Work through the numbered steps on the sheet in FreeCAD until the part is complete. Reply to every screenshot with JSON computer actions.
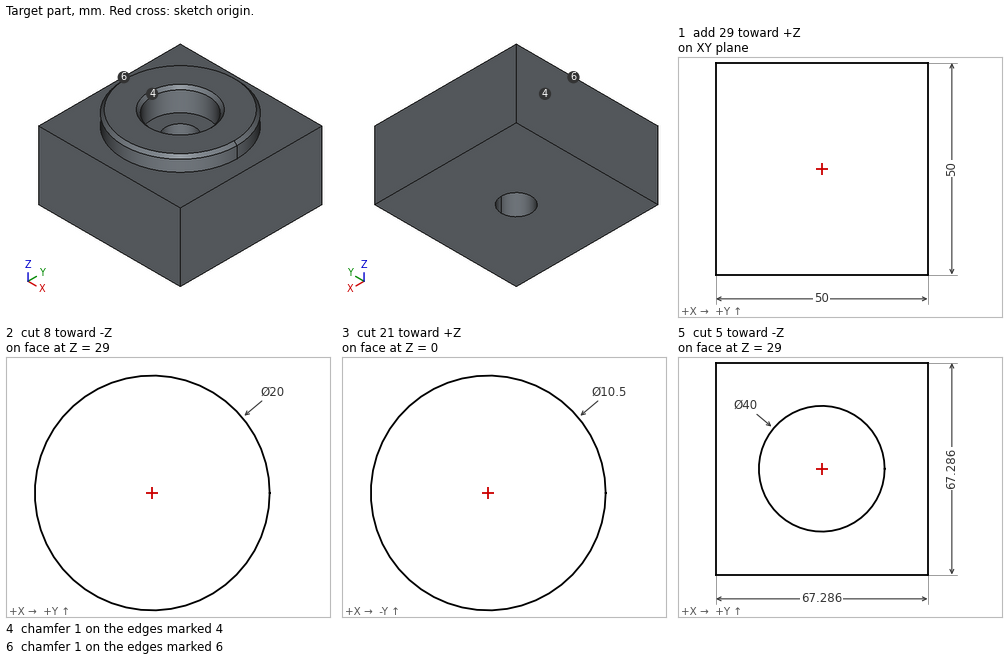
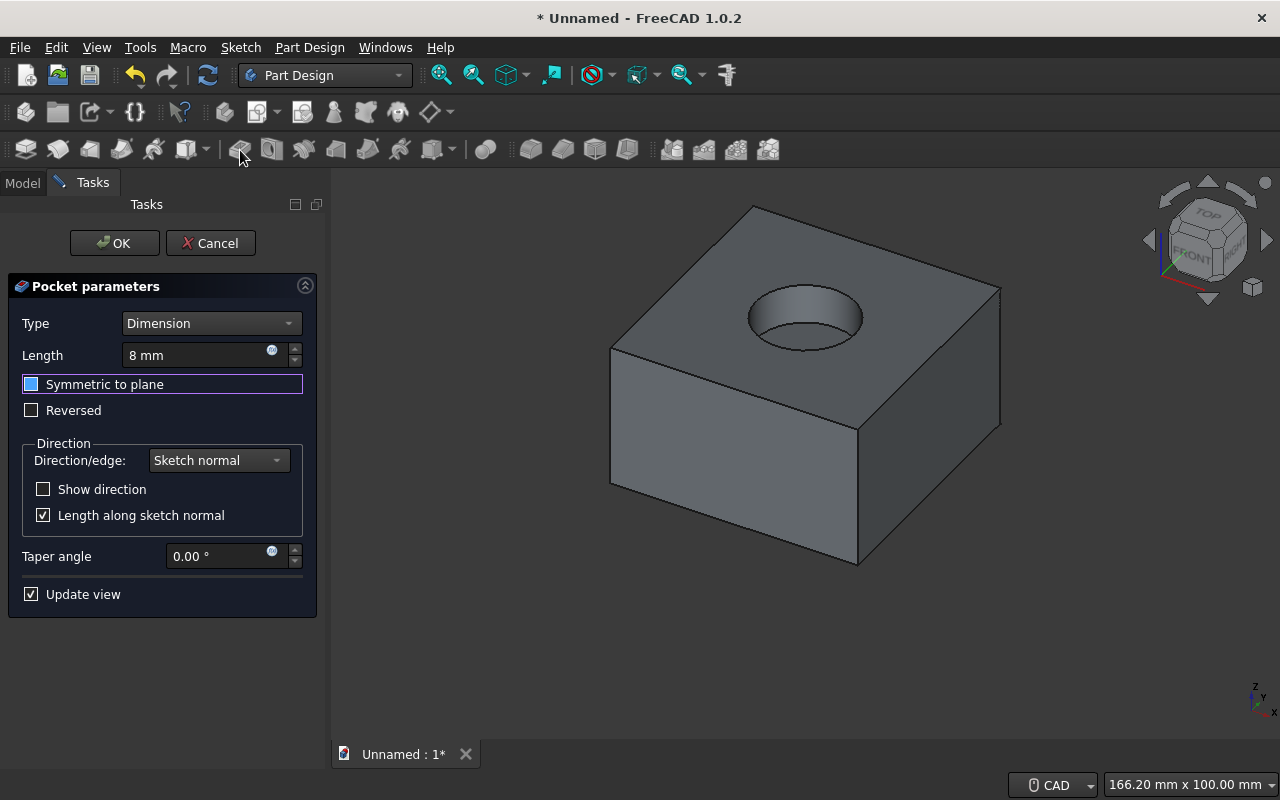
{"action": "left_click", "coordinate": [115, 243]}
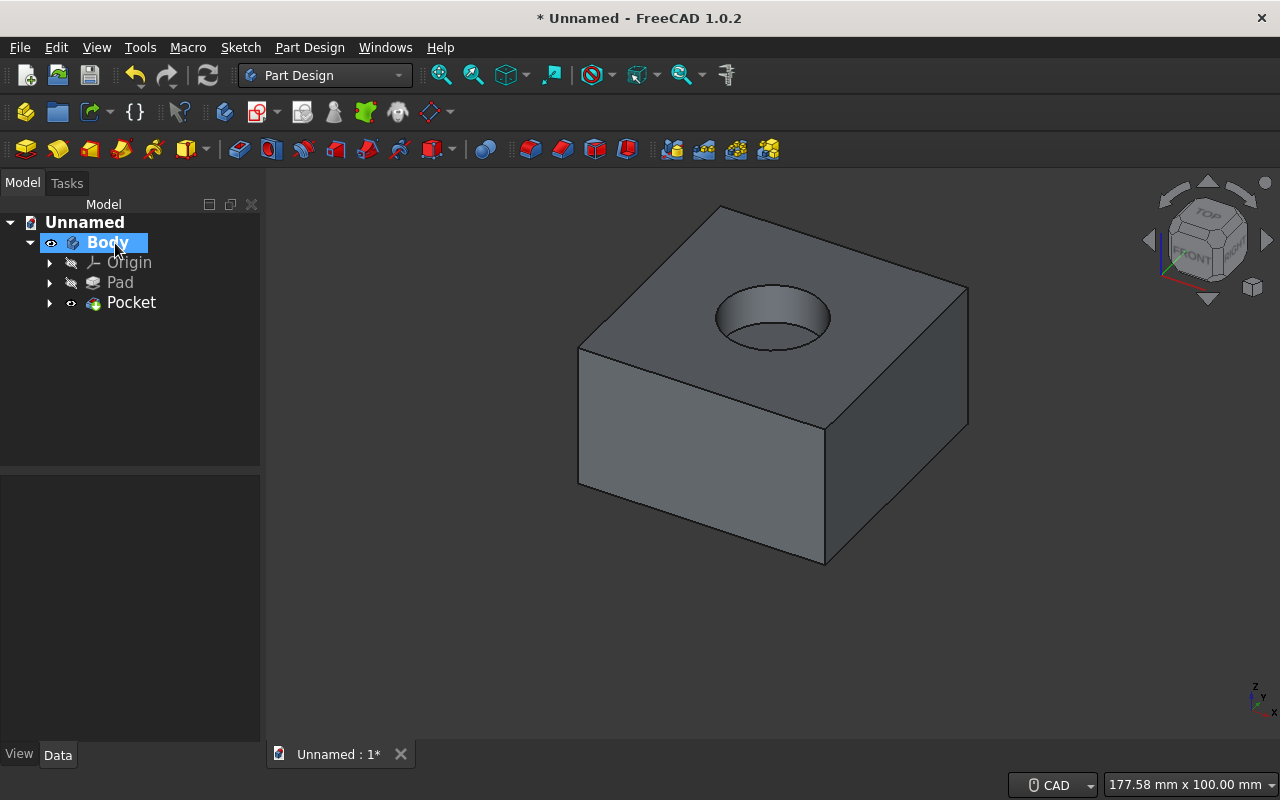
{"action": "key", "text": "5"}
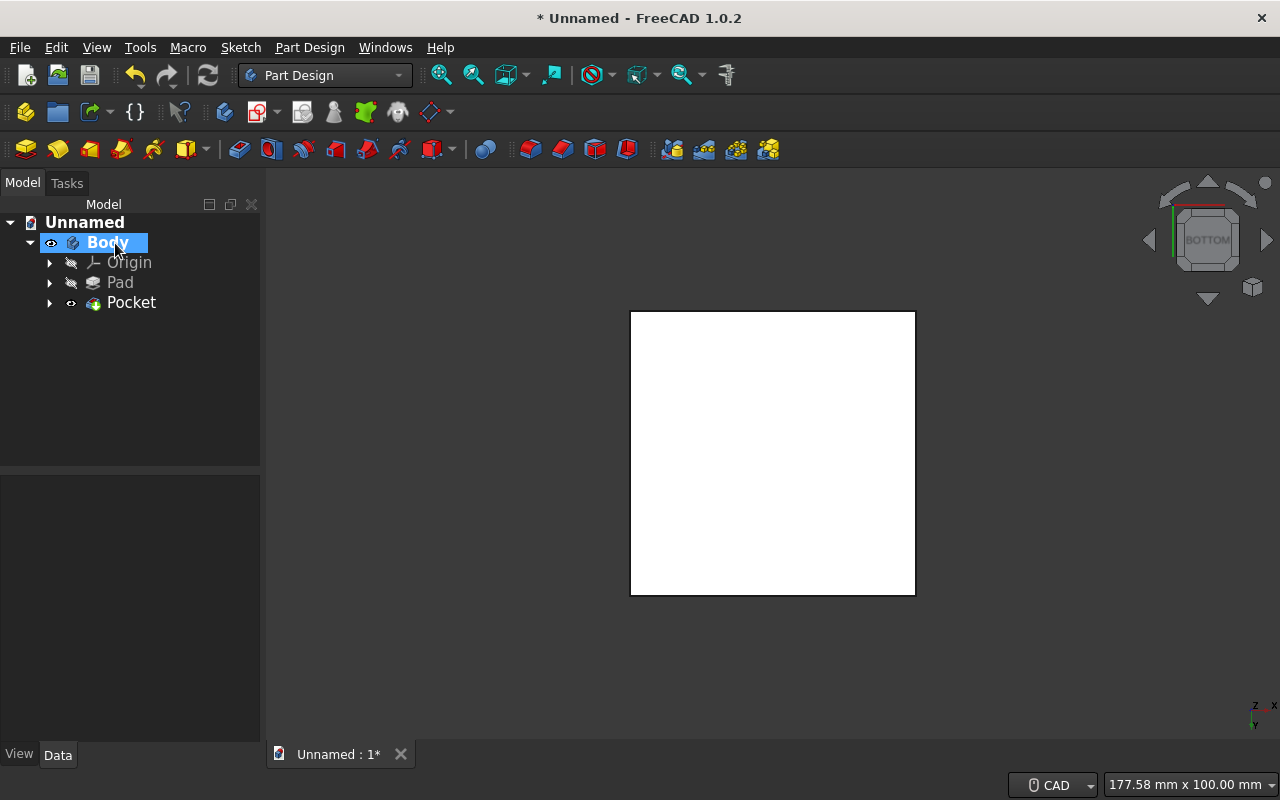
{"action": "left_click", "coordinate": [773, 452]}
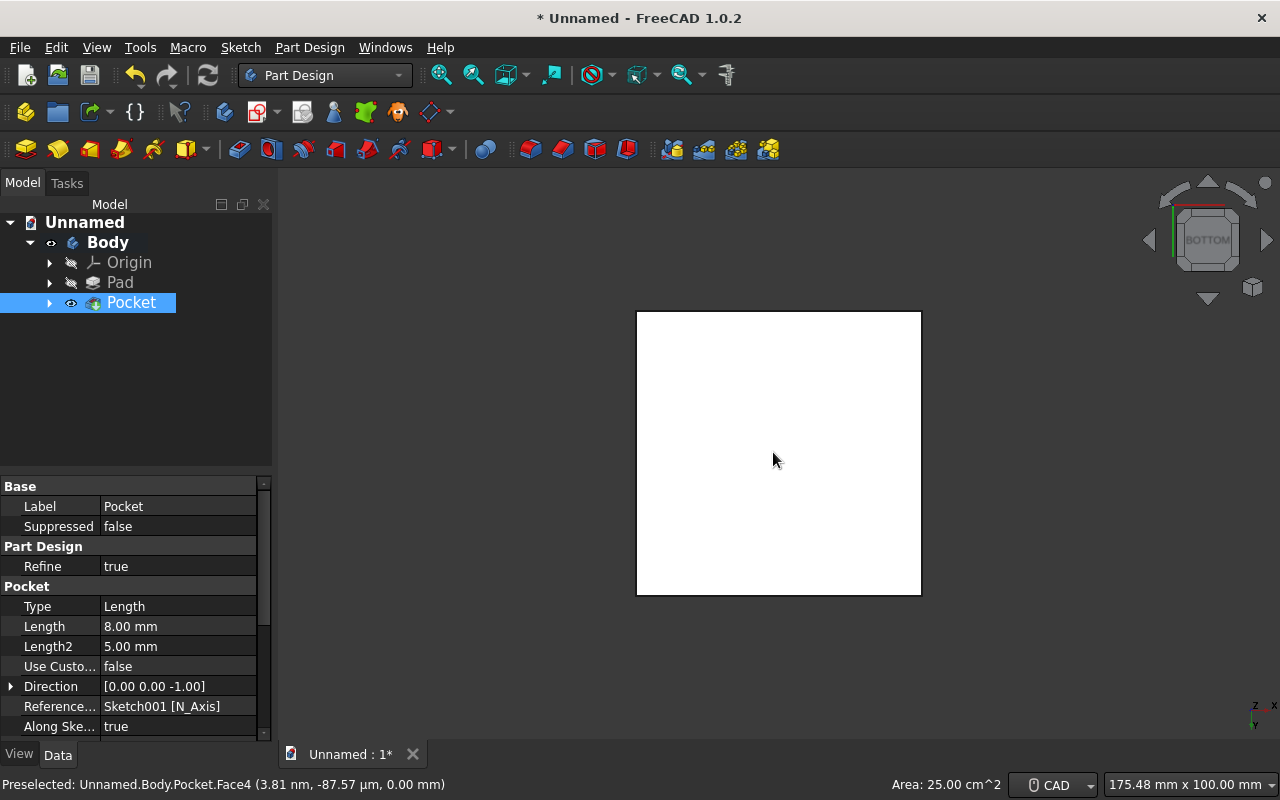
{"action": "left_click", "coordinate": [258, 112]}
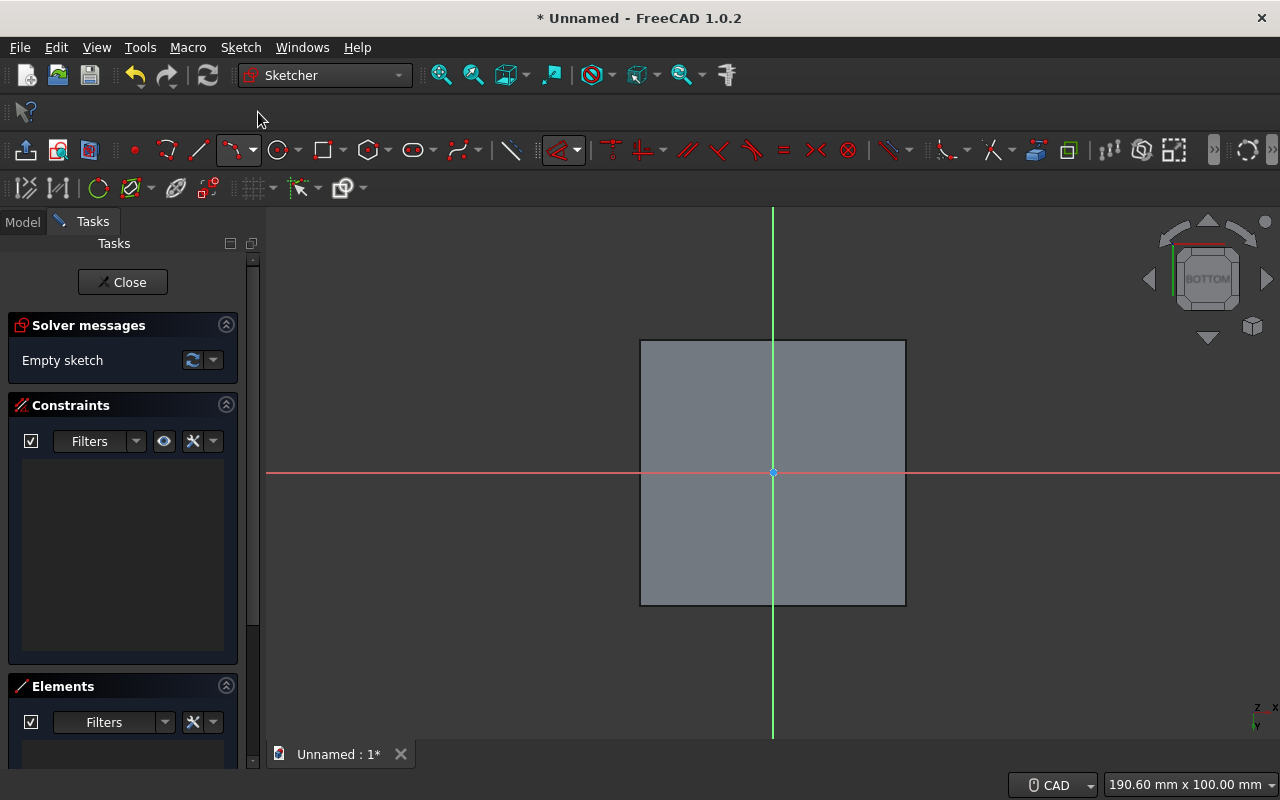
{"action": "scroll", "coordinate": [787, 473], "scroll_direction": "up", "scroll_amount": 9}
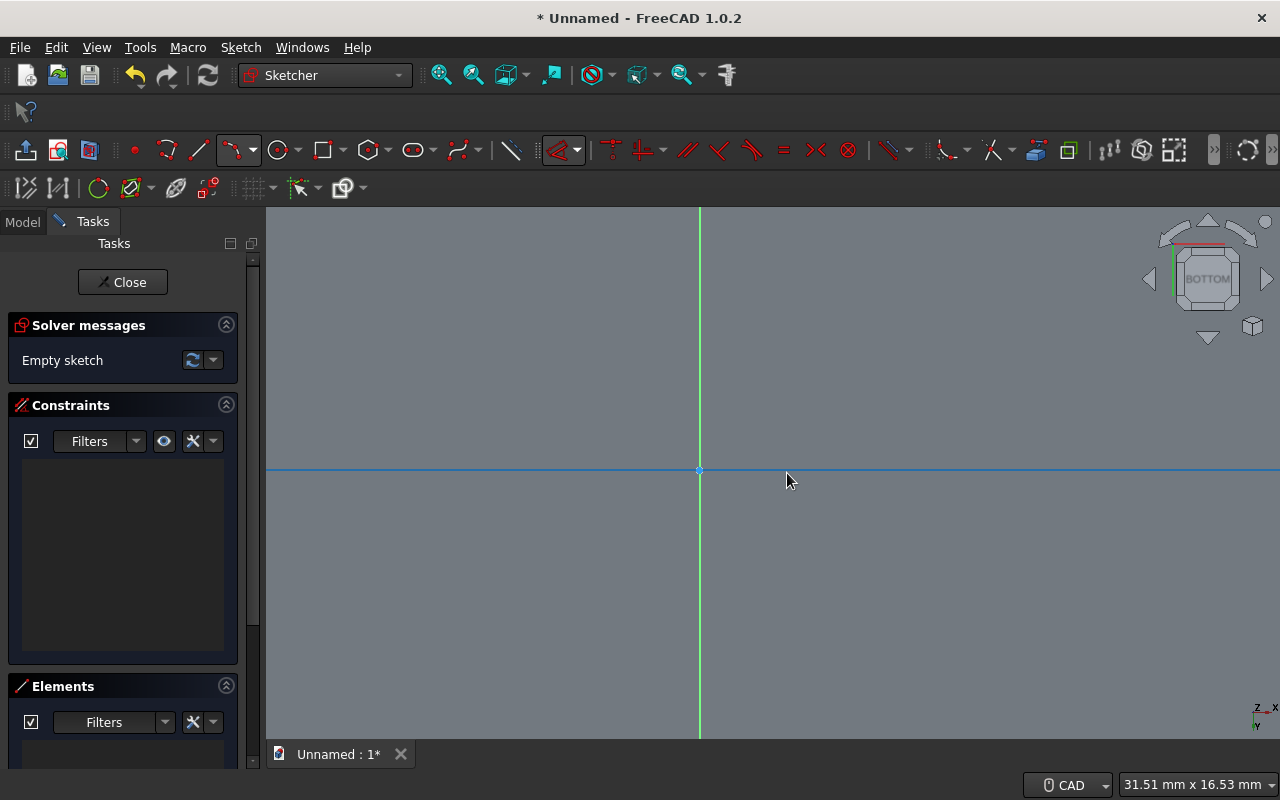
{"action": "left_click", "coordinate": [278, 150]}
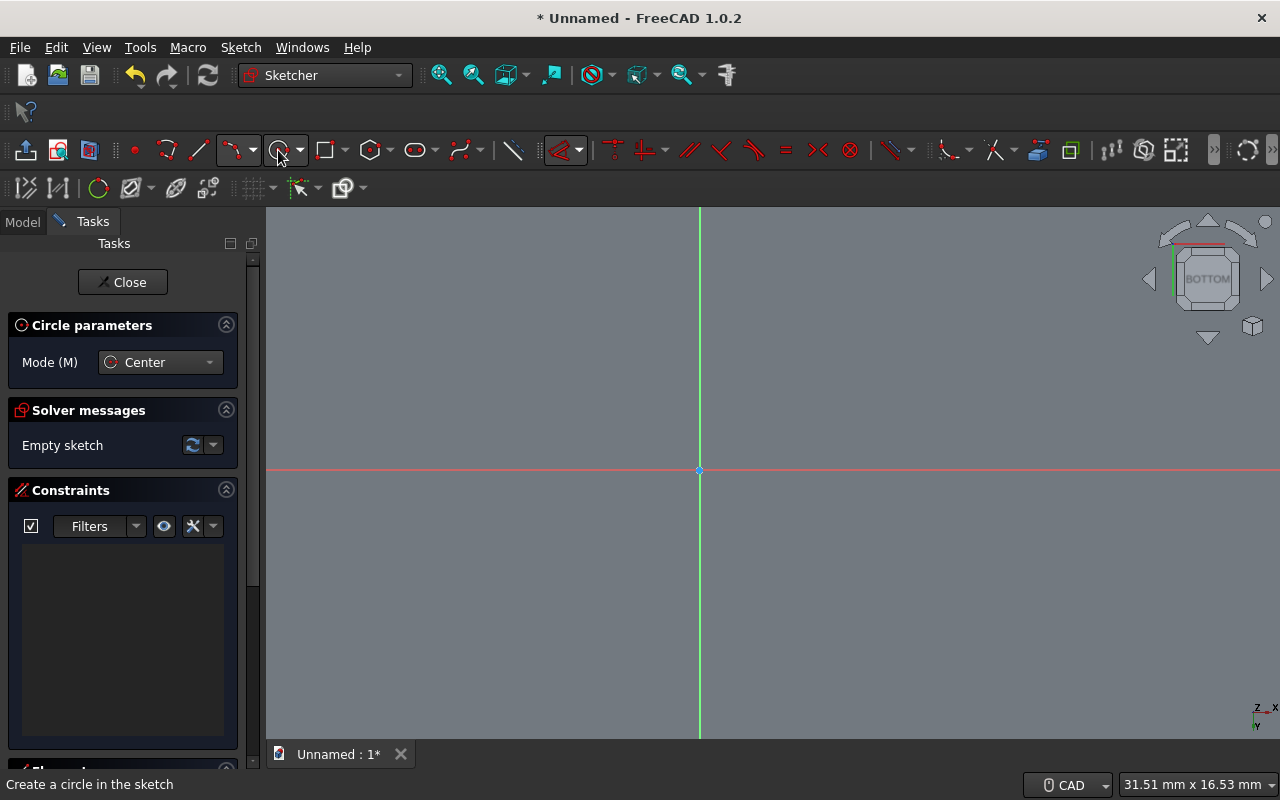
{"action": "left_click", "coordinate": [700, 470]}
{"action": "mouse_move", "coordinate": [819, 351]}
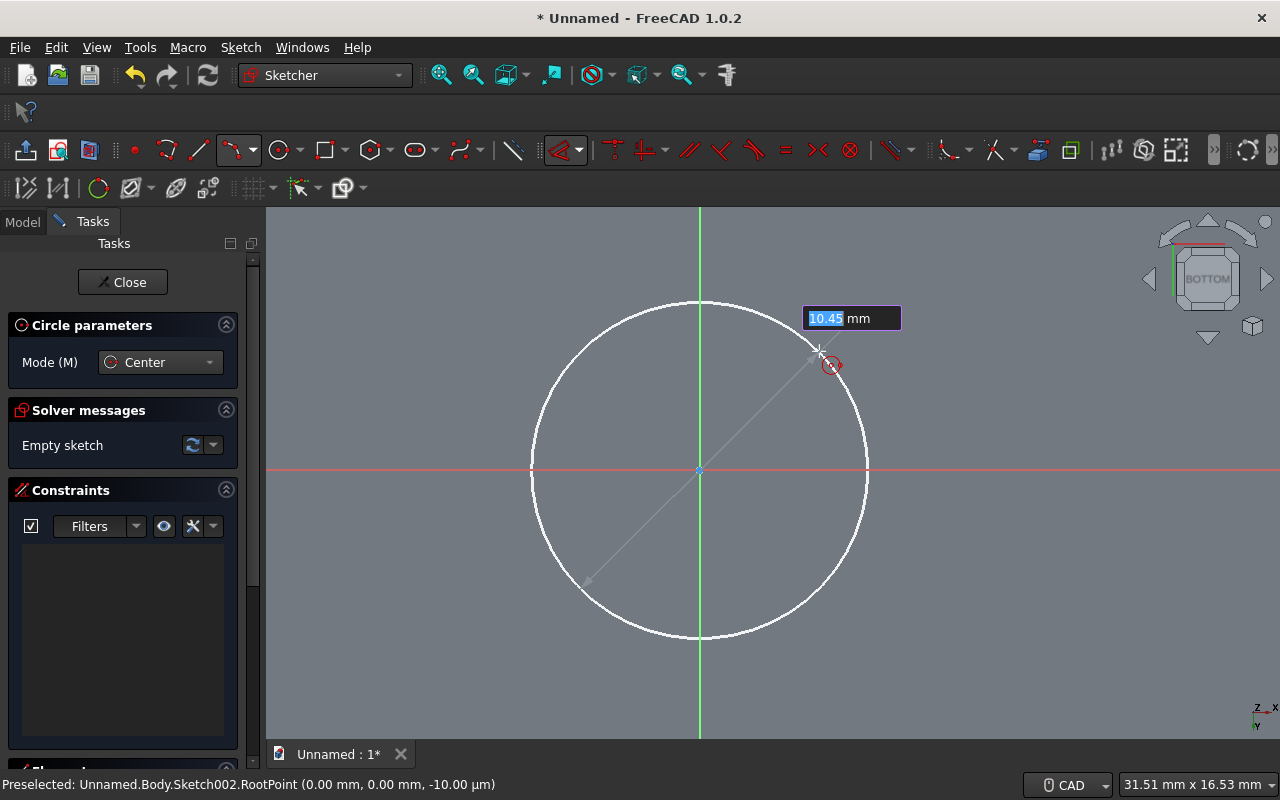
{"action": "type", "text": "10.5"}
{"action": "key", "text": "Return"}
{"action": "key", "text": "Escape"}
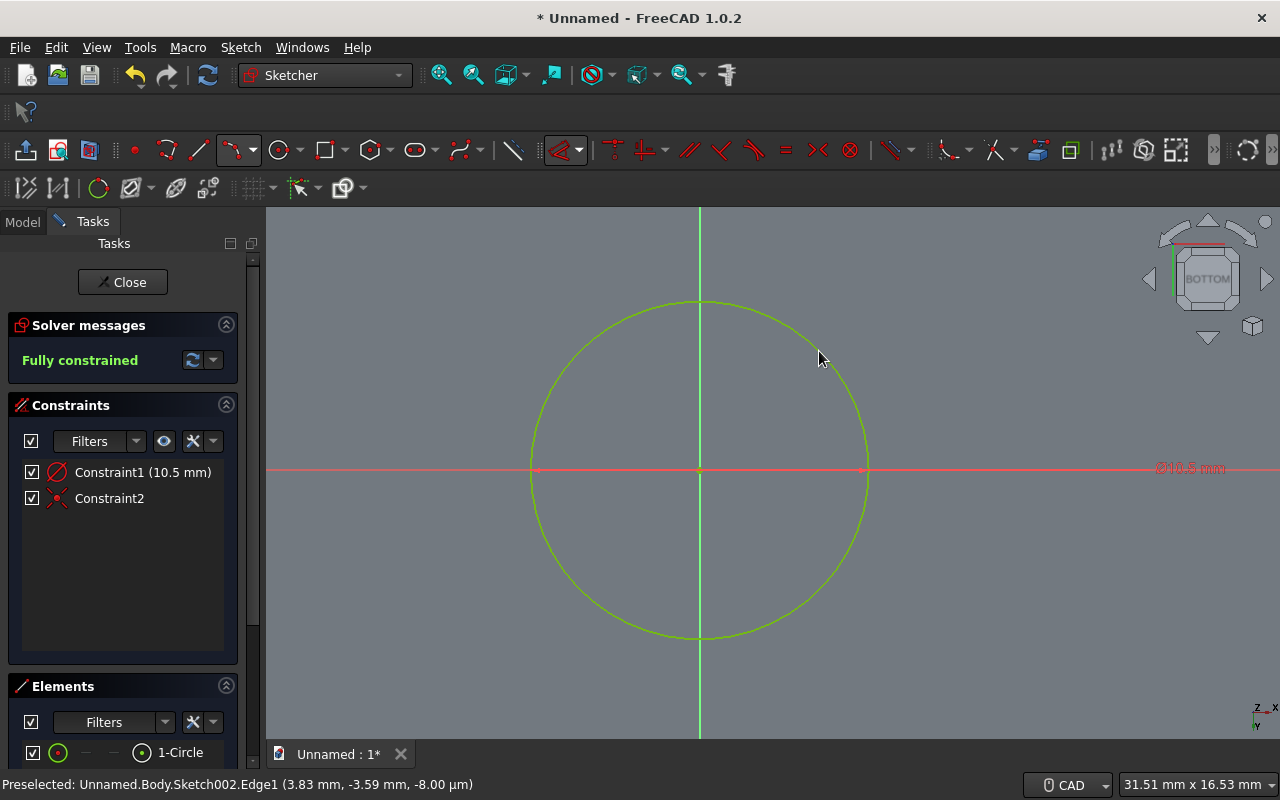
{"action": "left_click", "coordinate": [123, 282]}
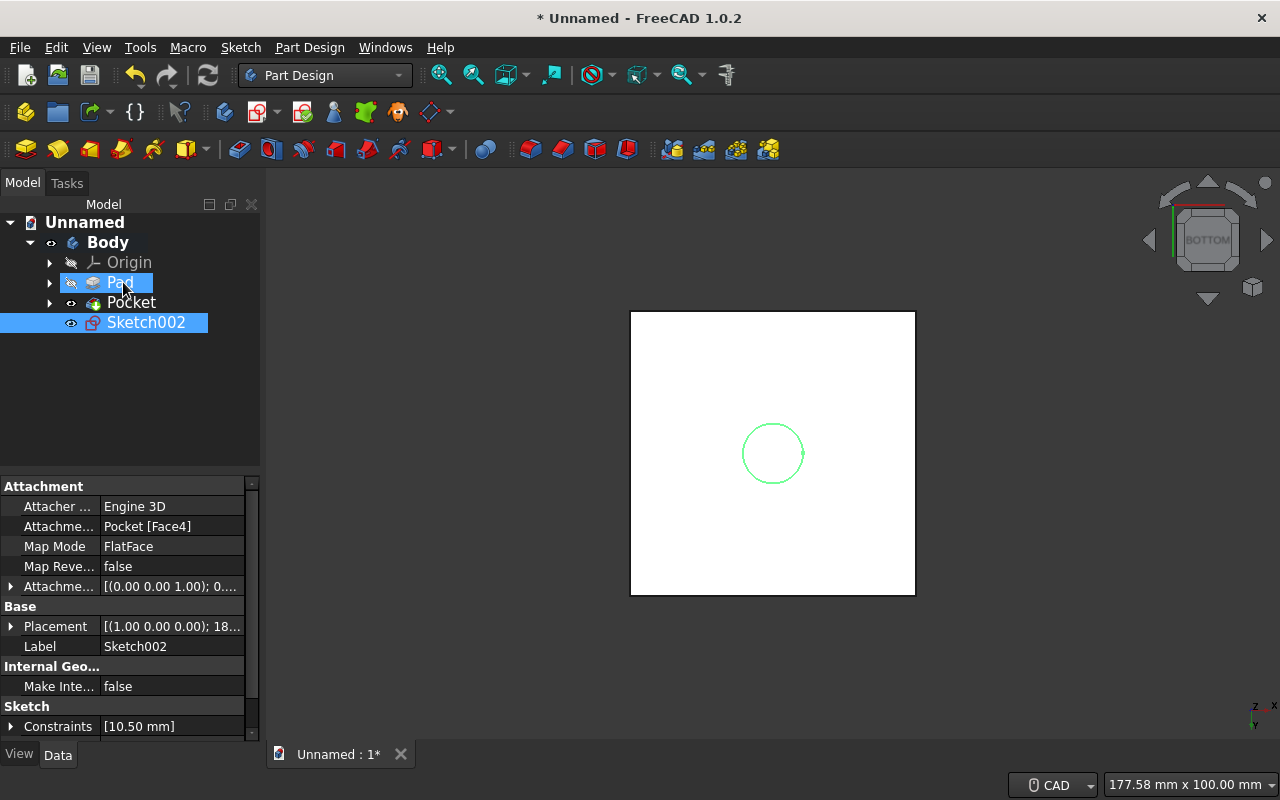
{"action": "left_click", "coordinate": [240, 150]}